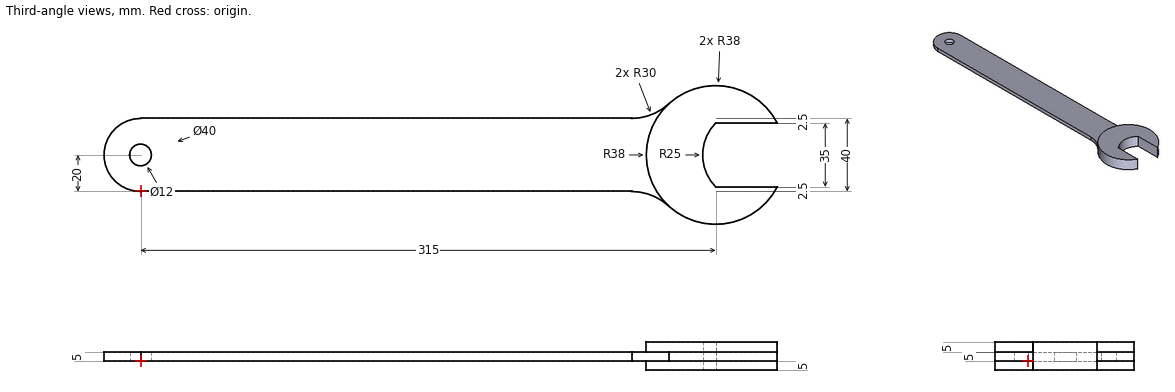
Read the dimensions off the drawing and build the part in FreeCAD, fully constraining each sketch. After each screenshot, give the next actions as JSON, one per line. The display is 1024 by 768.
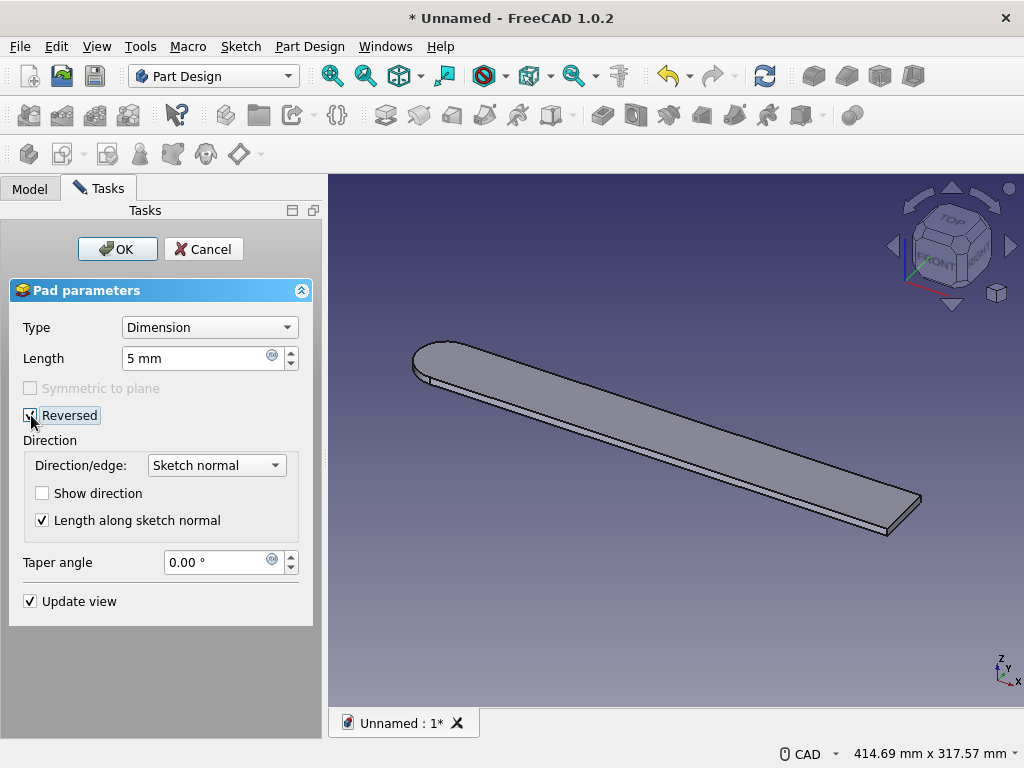
{"action": "left_click", "coordinate": [118, 249]}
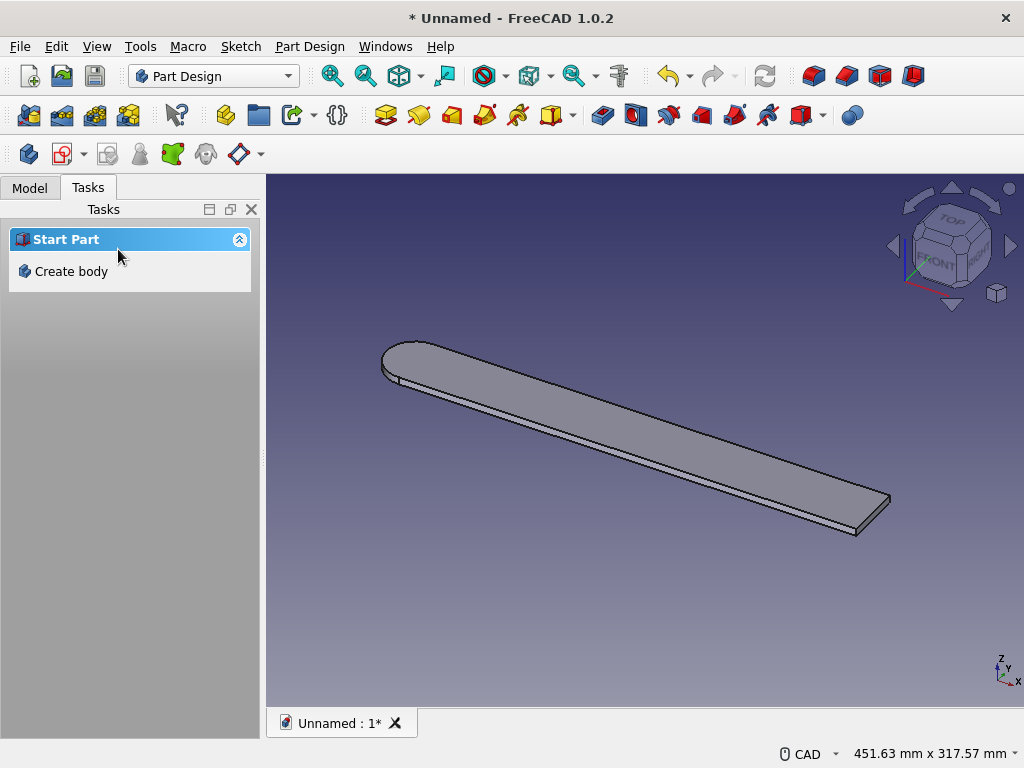
{"action": "left_click", "coordinate": [838, 500]}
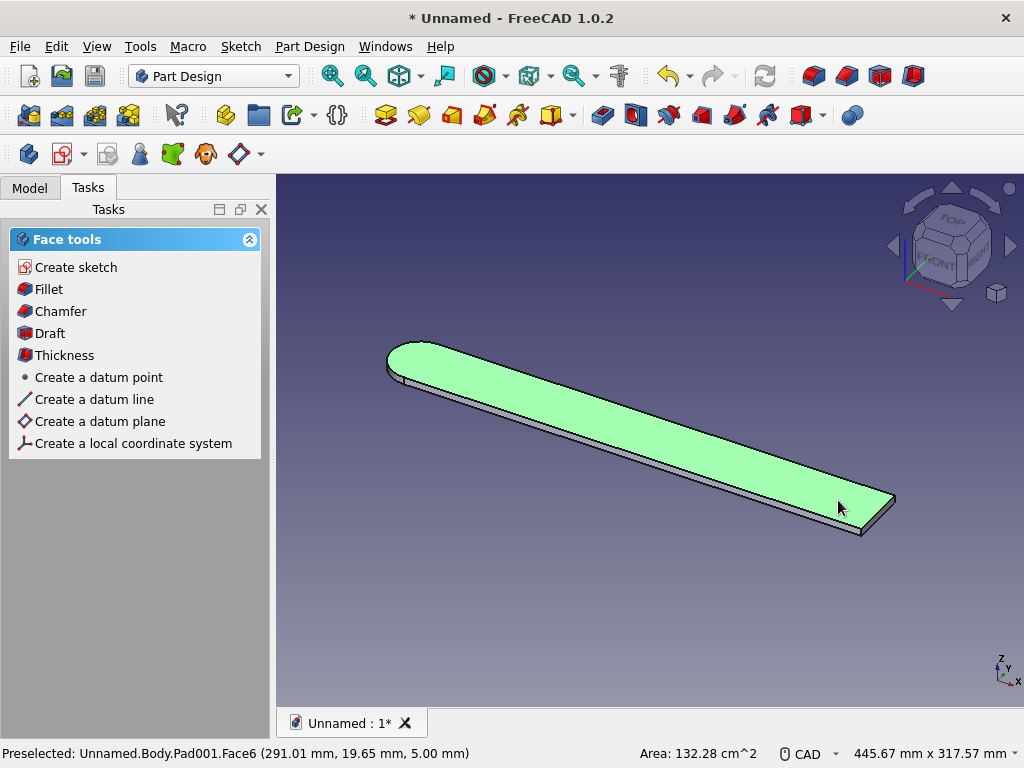
{"action": "left_click", "coordinate": [62, 154]}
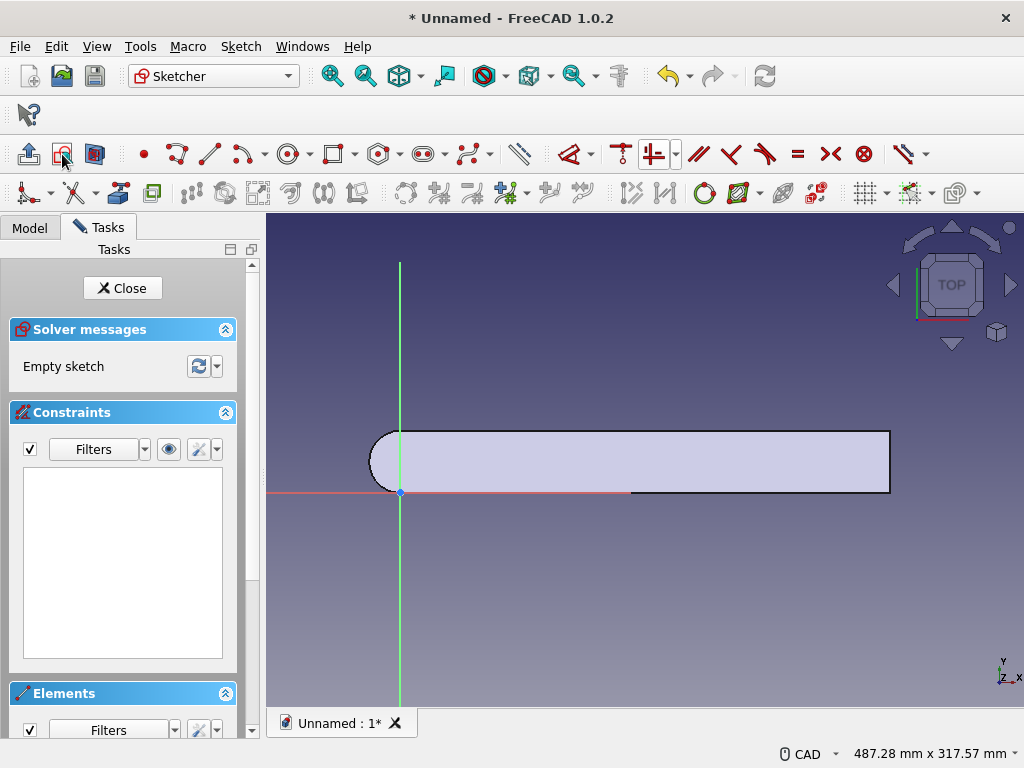
{"action": "scroll", "coordinate": [576, 460], "scroll_direction": "down", "scroll_amount": 5}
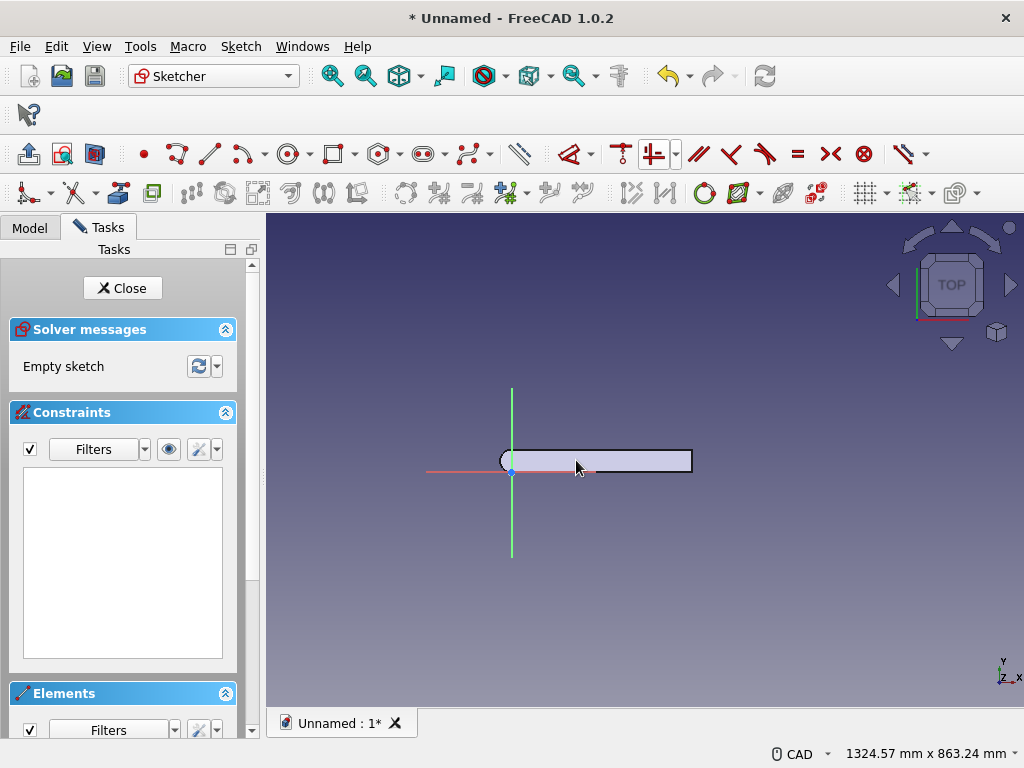
{"action": "scroll", "coordinate": [710, 461], "scroll_direction": "up", "scroll_amount": 10}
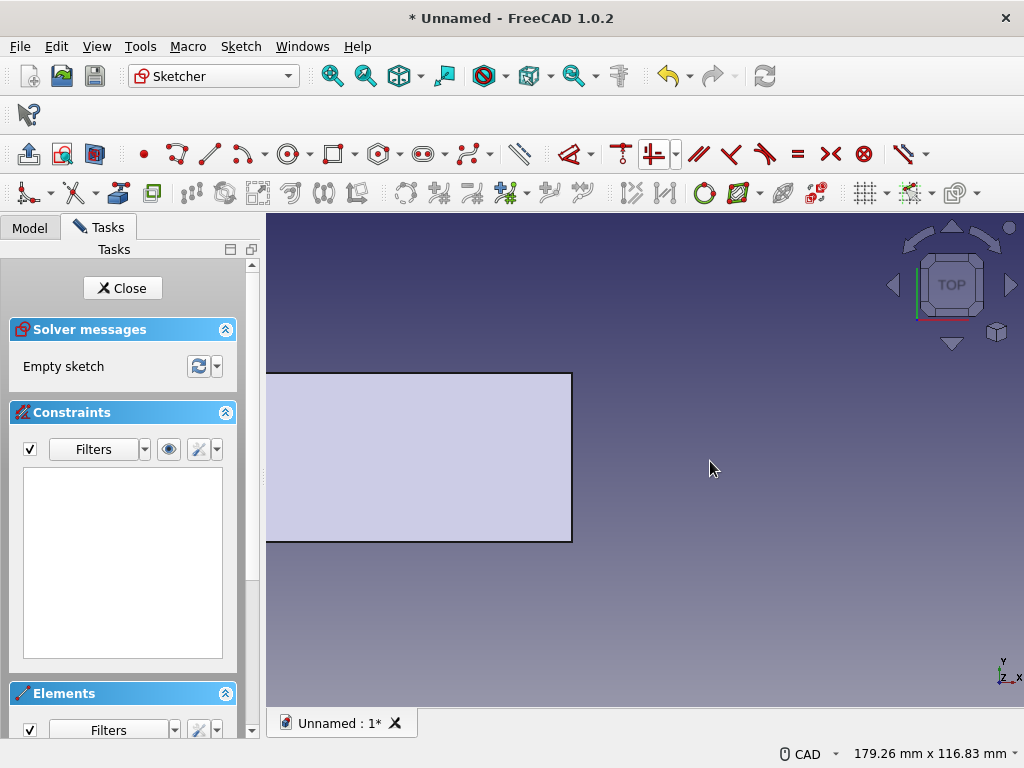
{"action": "left_click", "coordinate": [177, 154]}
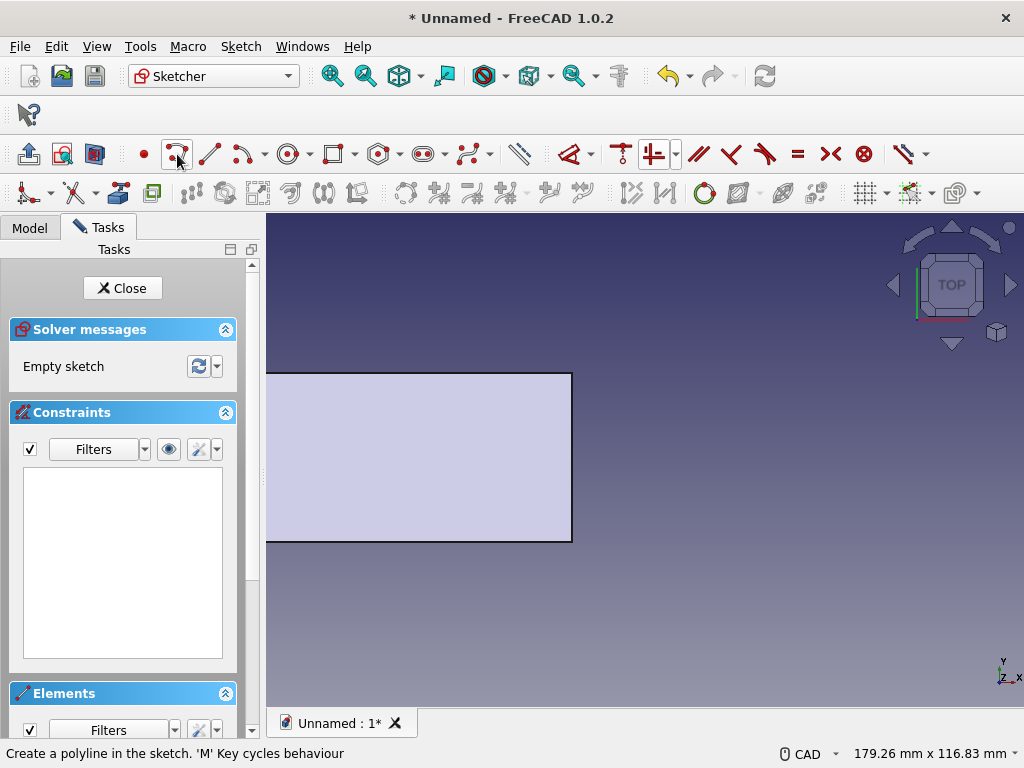
{"action": "left_click", "coordinate": [436, 373]}
{"action": "left_click", "coordinate": [572, 373]}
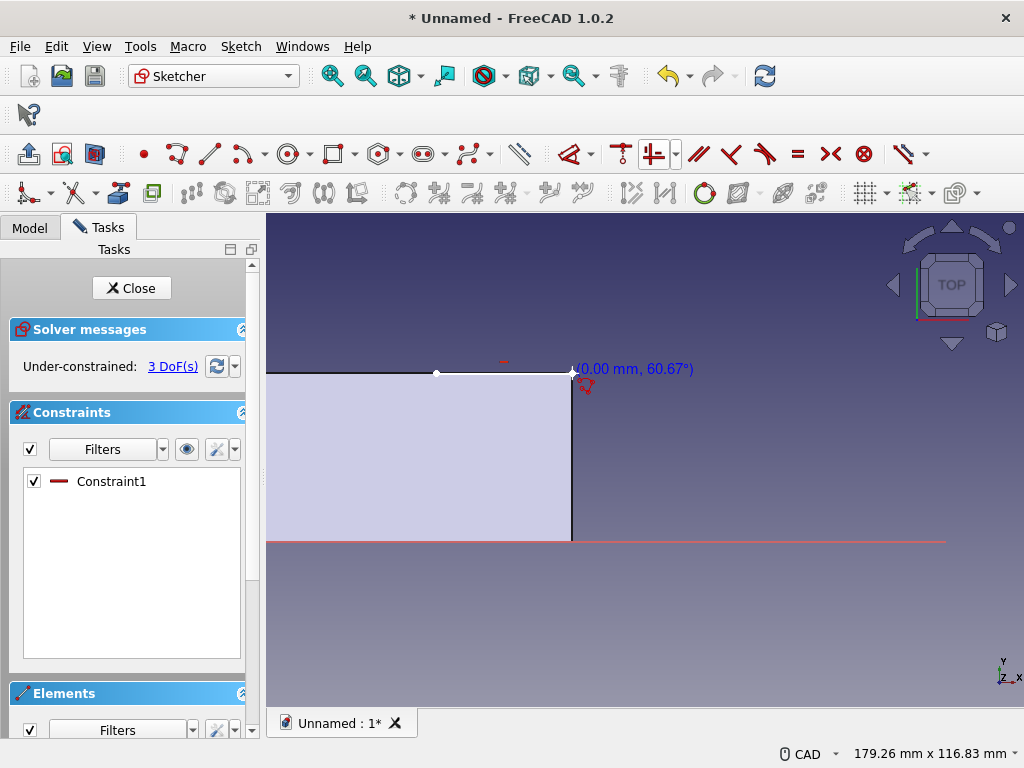
{"action": "scroll", "coordinate": [572, 384], "scroll_direction": "up", "scroll_amount": 3}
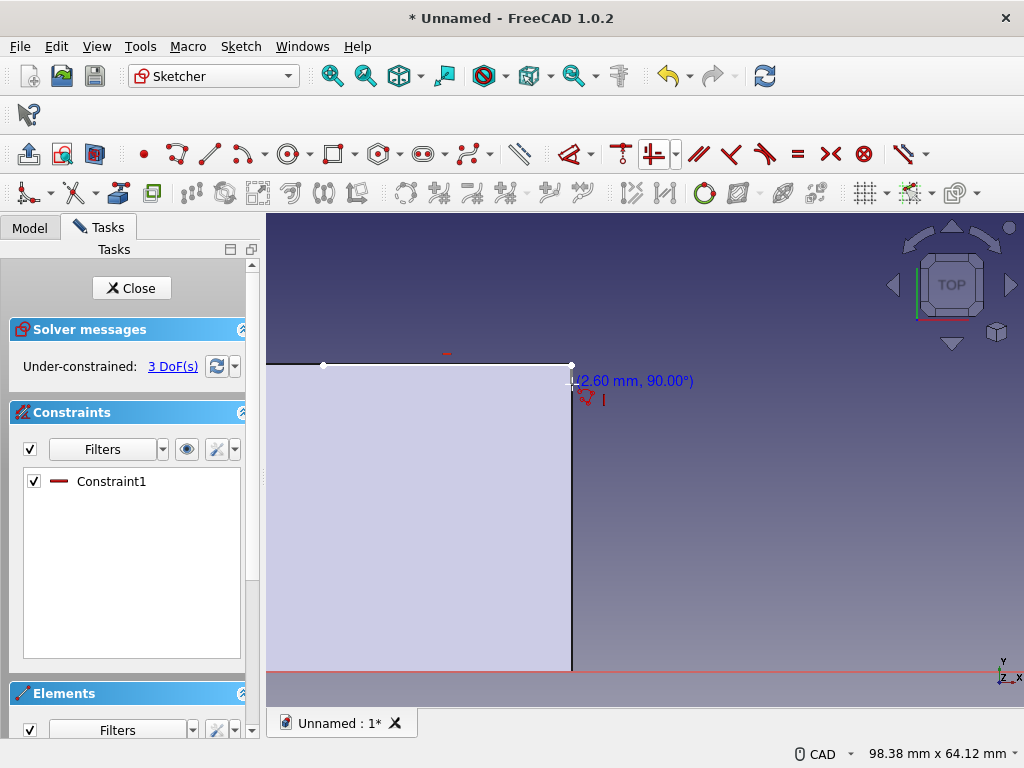
{"action": "left_click", "coordinate": [572, 383]}
{"action": "left_click", "coordinate": [832, 383]}
{"action": "right_click", "coordinate": [832, 383]}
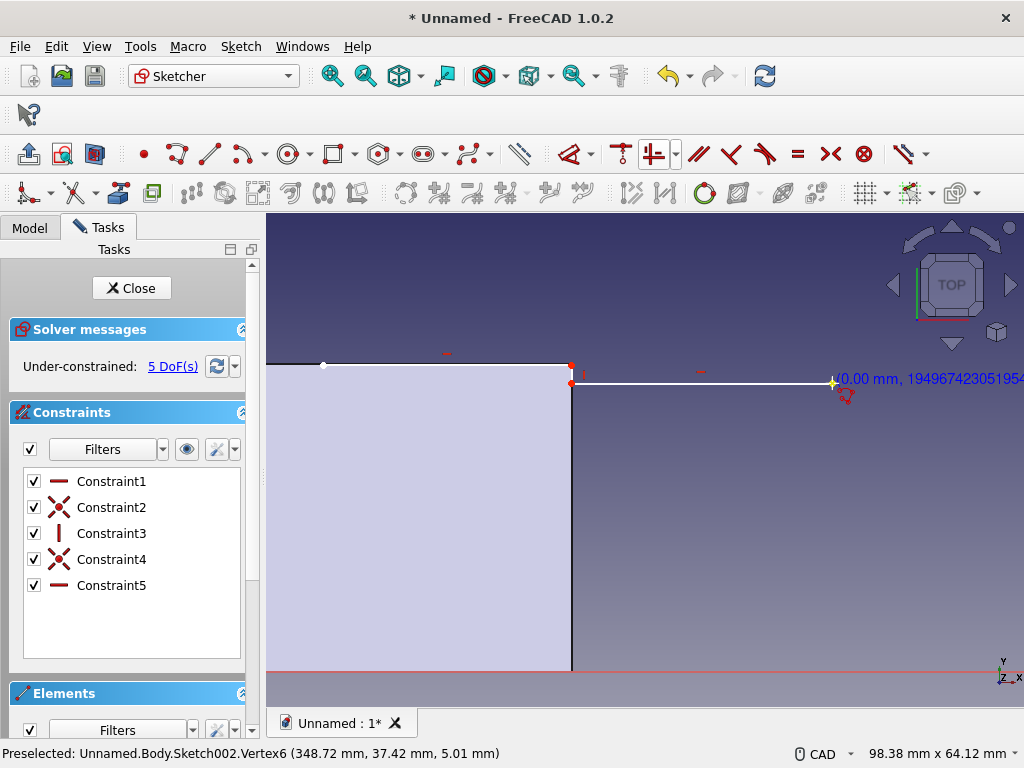
{"action": "key", "text": "g 3 a"}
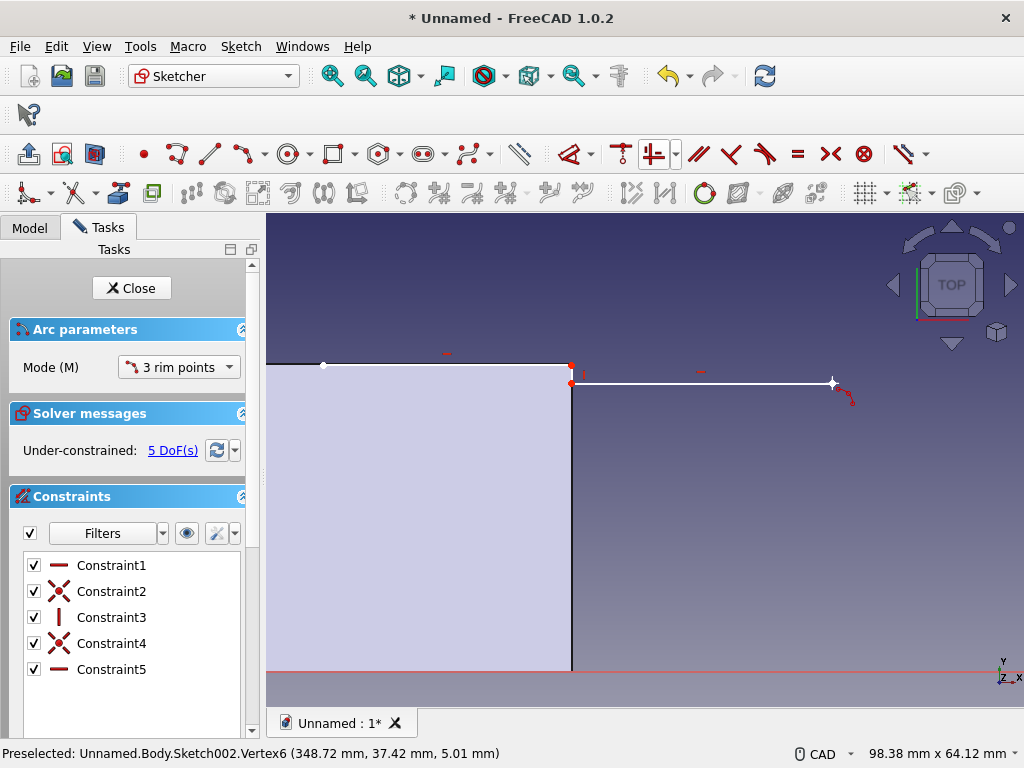
{"action": "left_click", "coordinate": [832, 384]}
{"action": "left_click", "coordinate": [324, 365]}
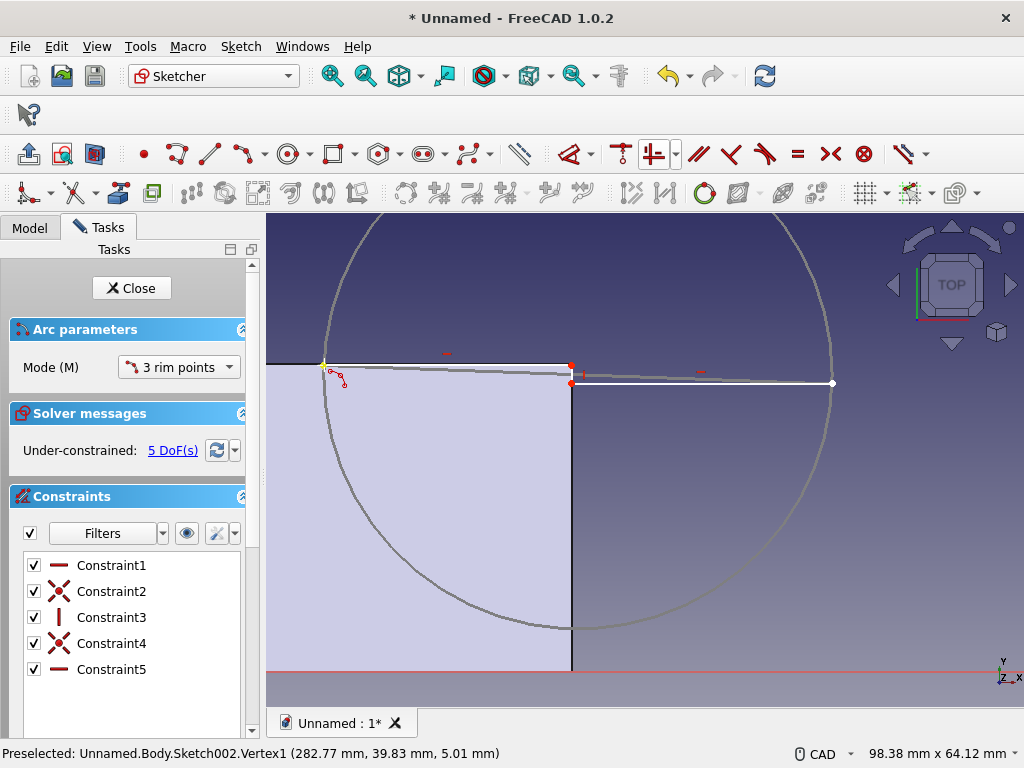
{"action": "scroll", "coordinate": [575, 389], "scroll_direction": "down", "scroll_amount": 3}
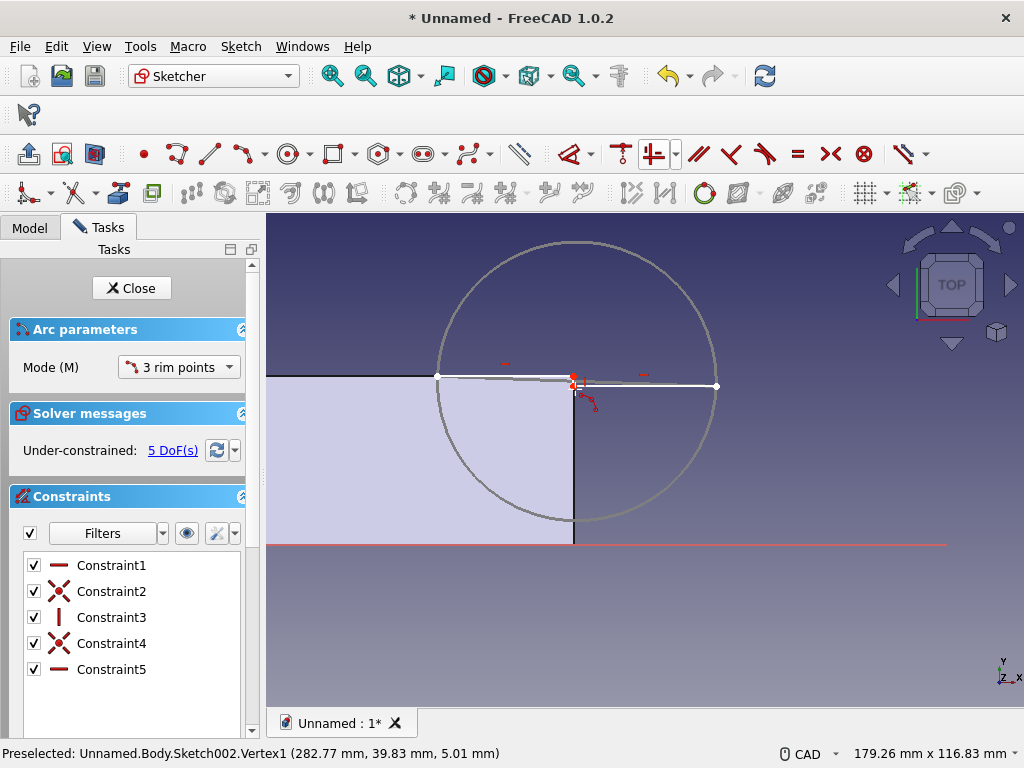
{"action": "left_click", "coordinate": [580, 300]}